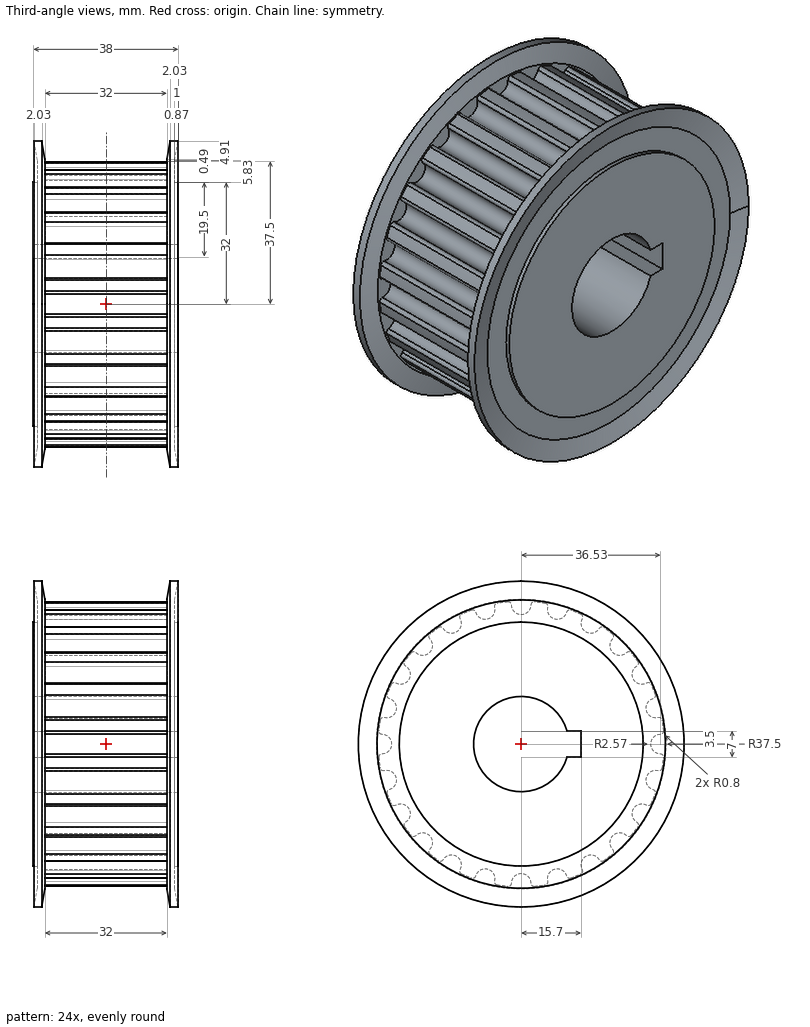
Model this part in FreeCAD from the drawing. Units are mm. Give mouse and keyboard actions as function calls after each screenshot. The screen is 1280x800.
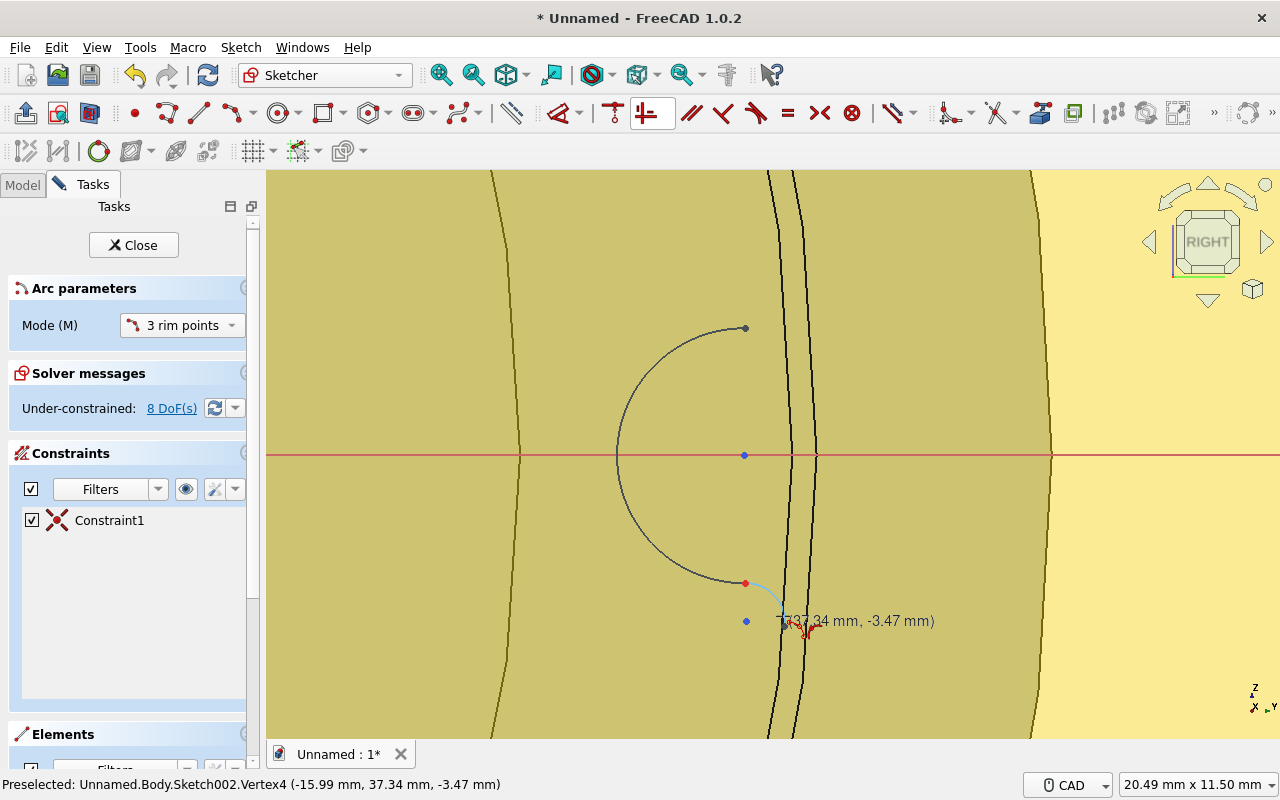
click(785, 284)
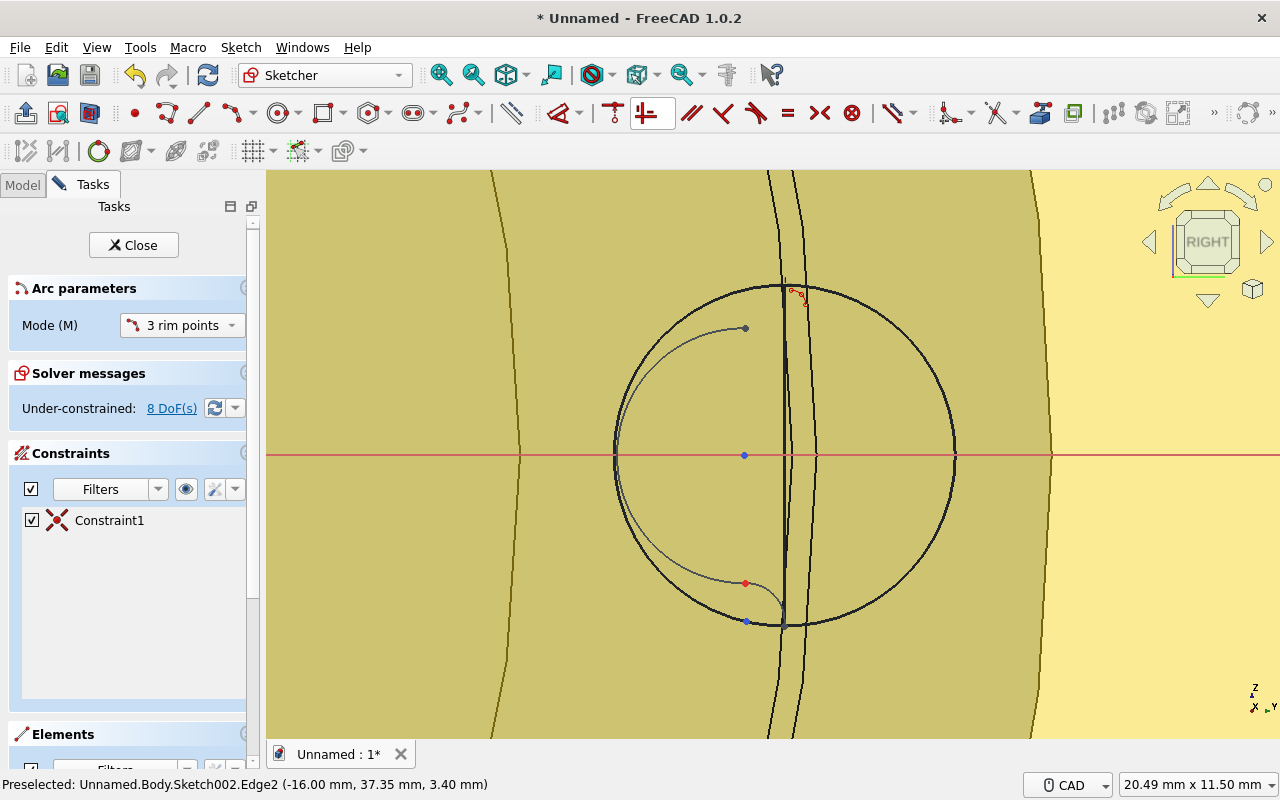
scroll(792, 489, up, 4)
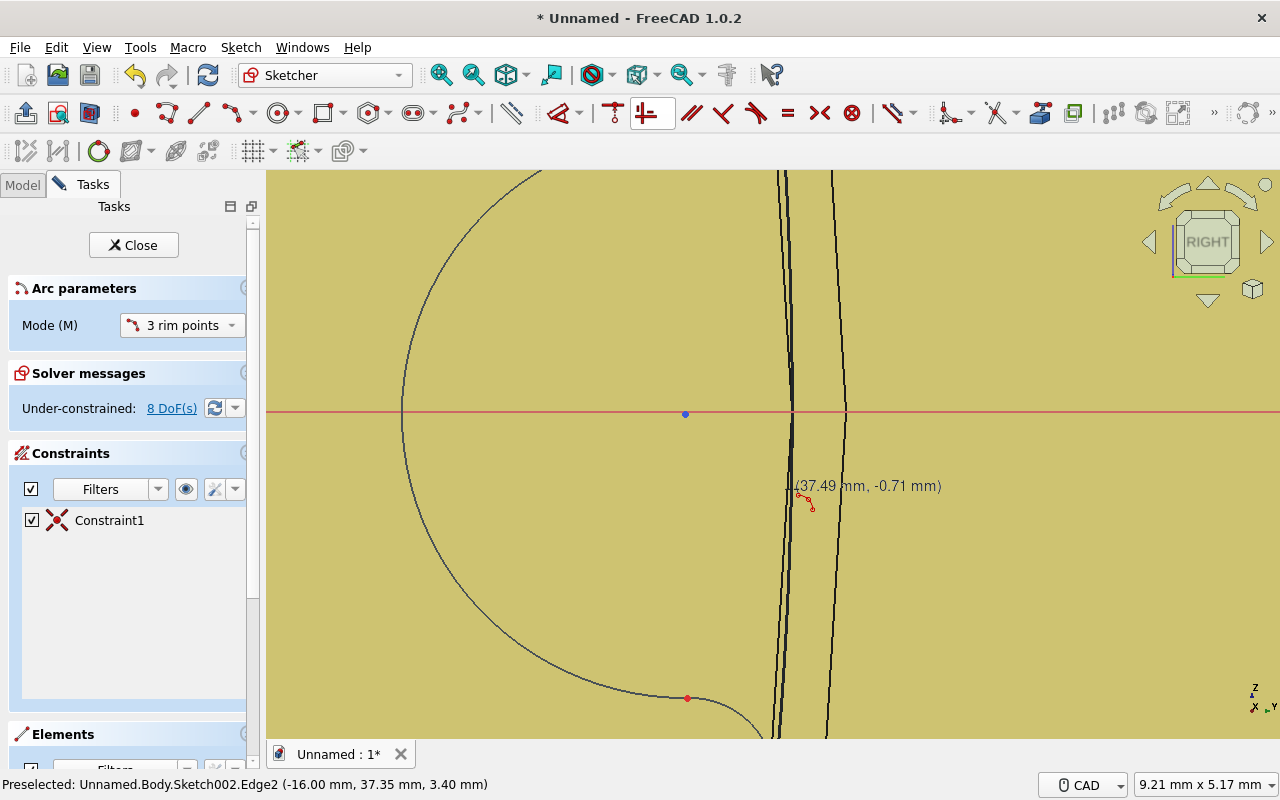
click(791, 488)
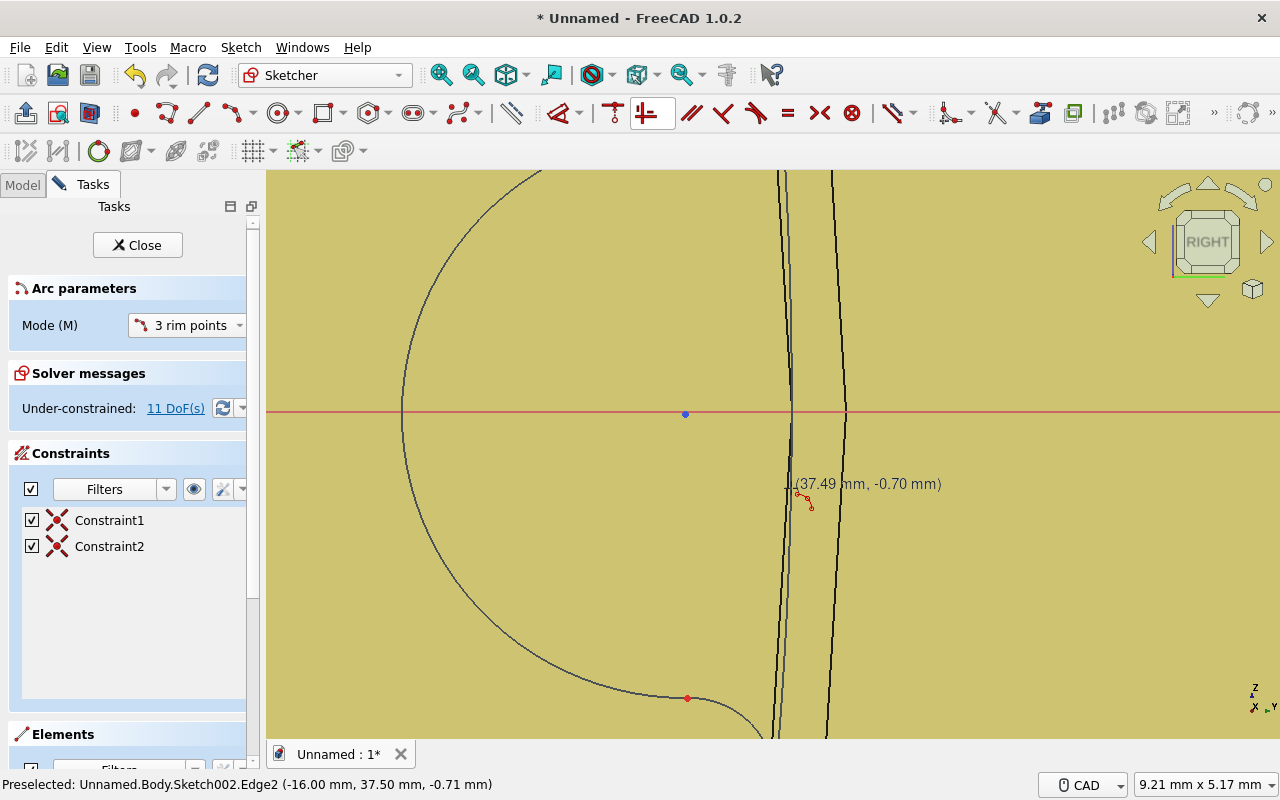
scroll(792, 489, down, 4)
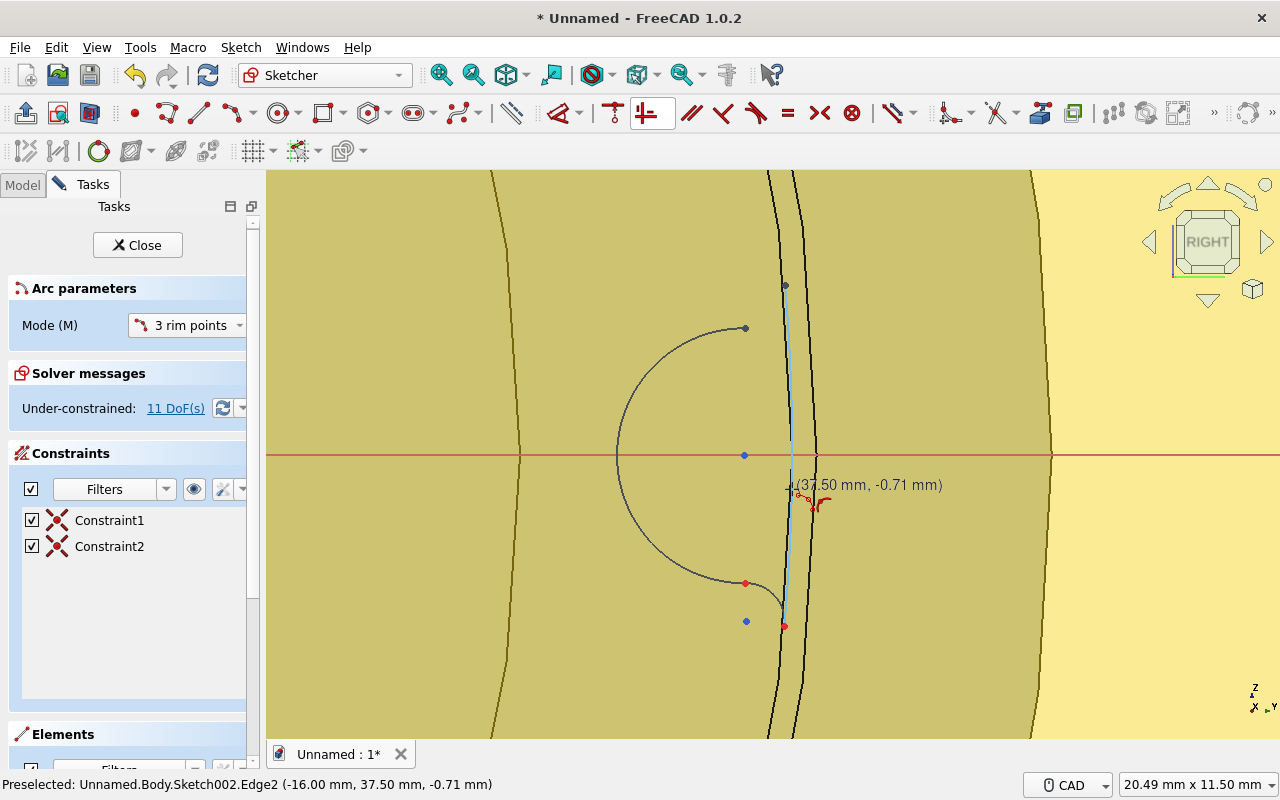
click(785, 285)
click(745, 328)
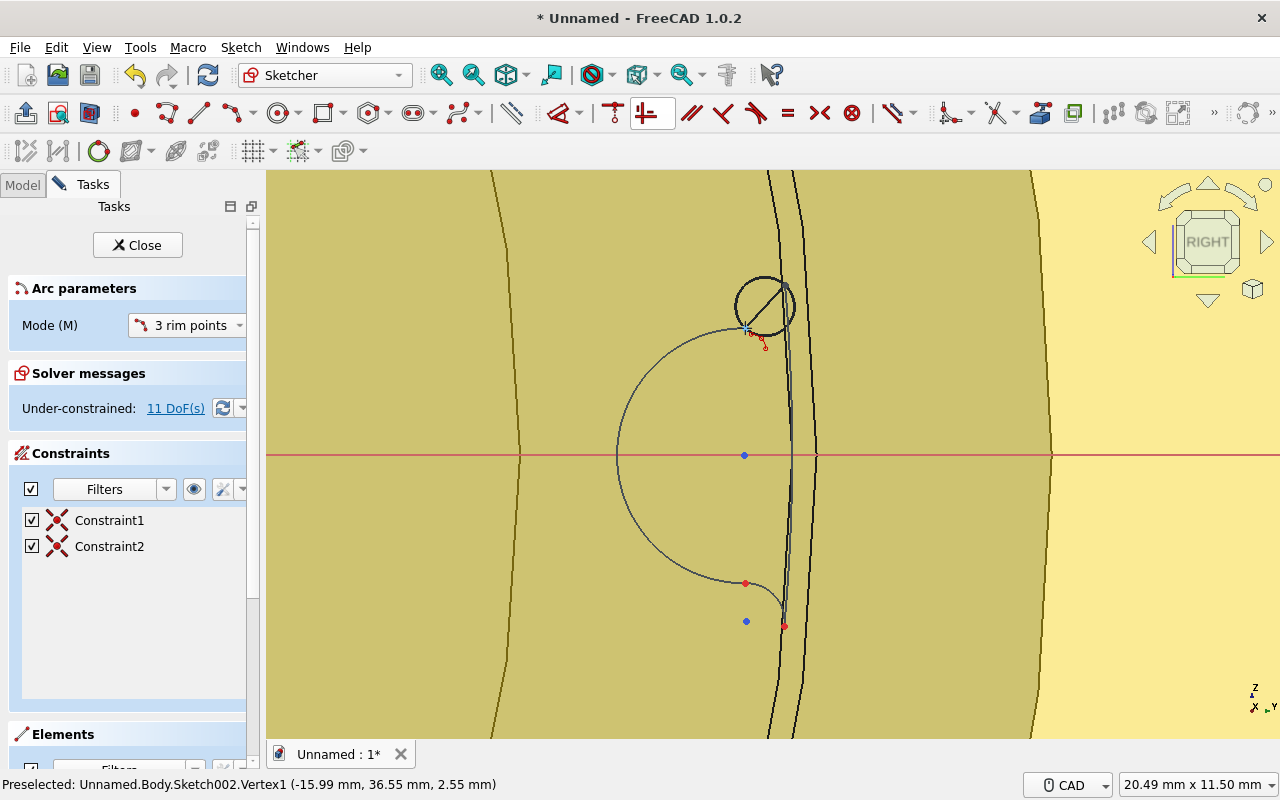
scroll(774, 315, up, 2)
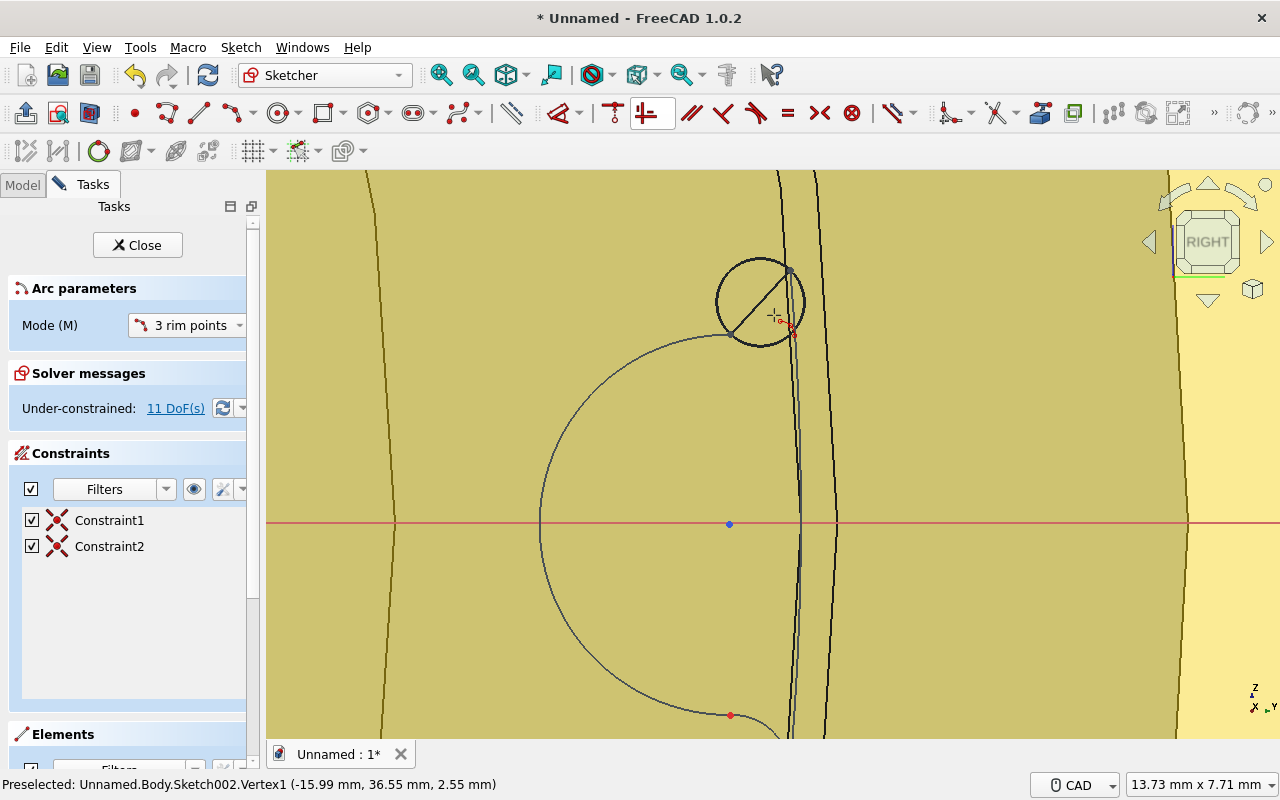
click(774, 314)
key(Escape)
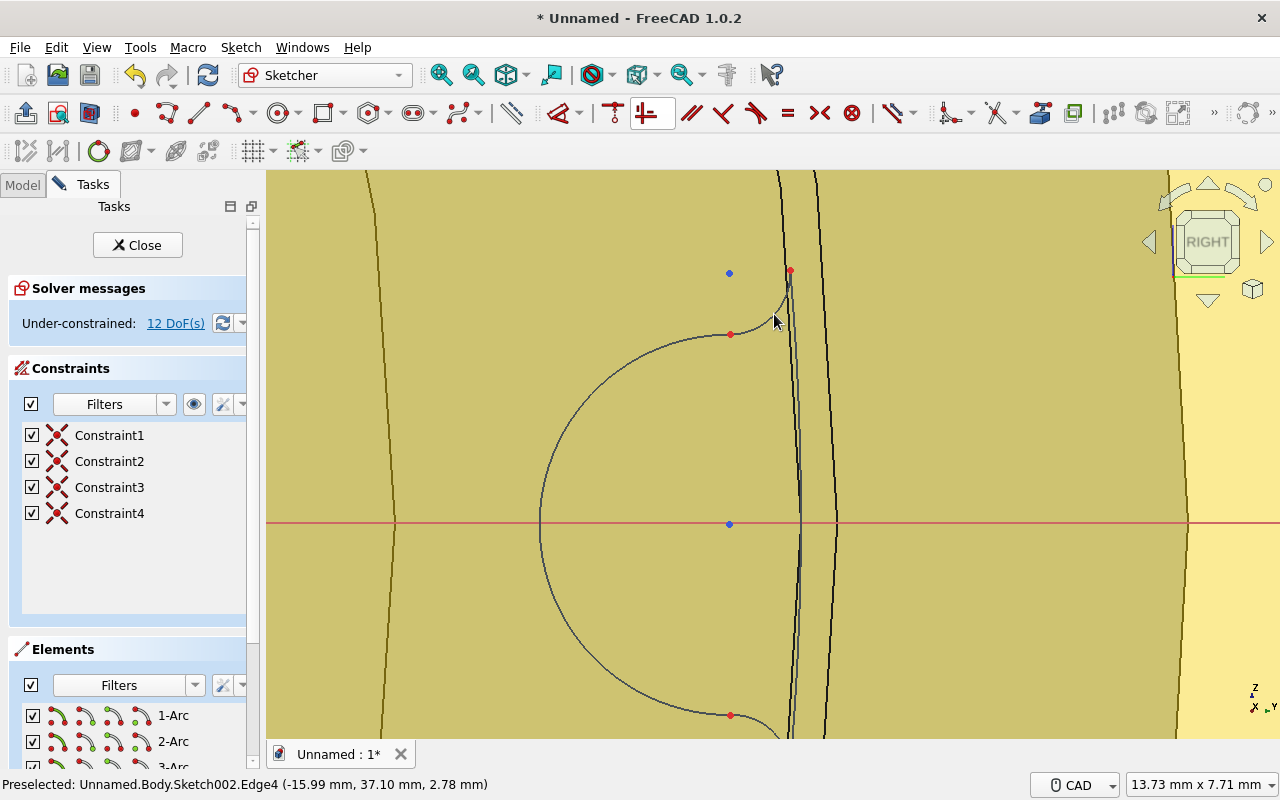
click(576, 413)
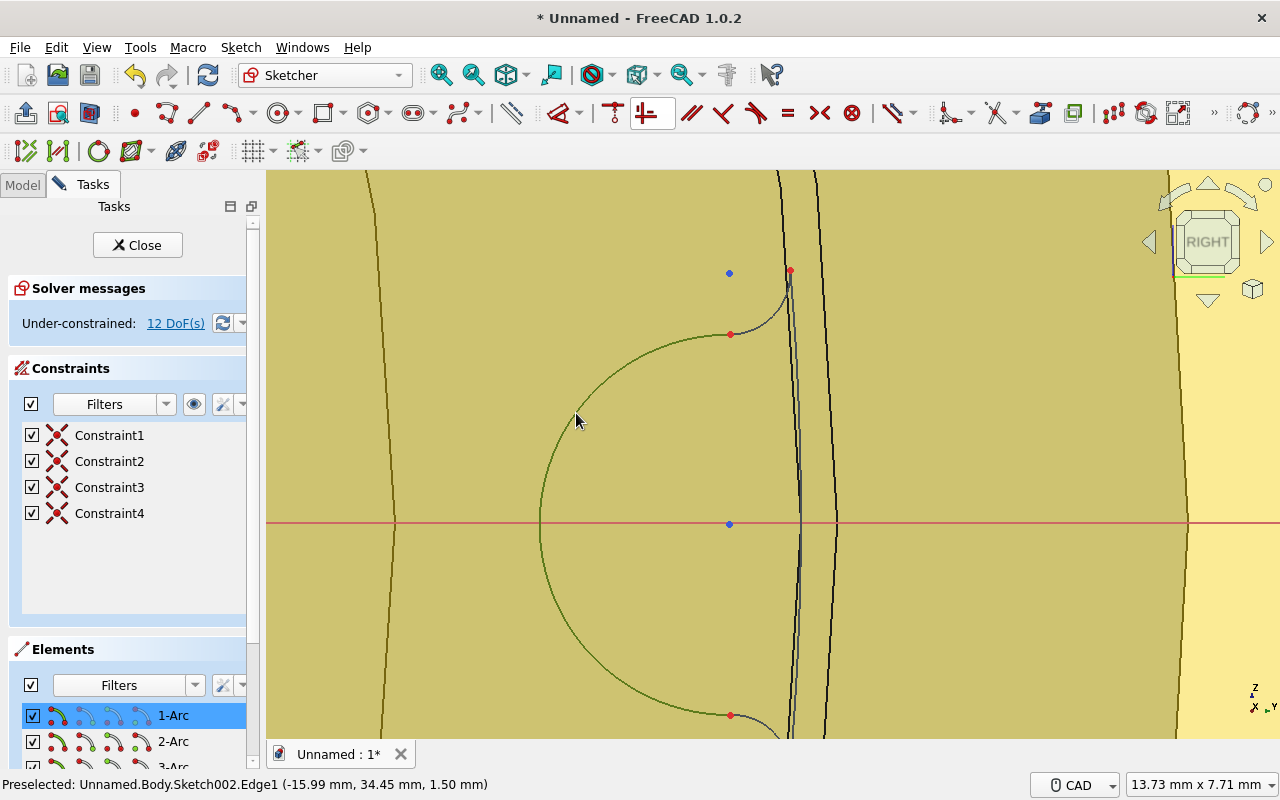
scroll(774, 315, down, 2)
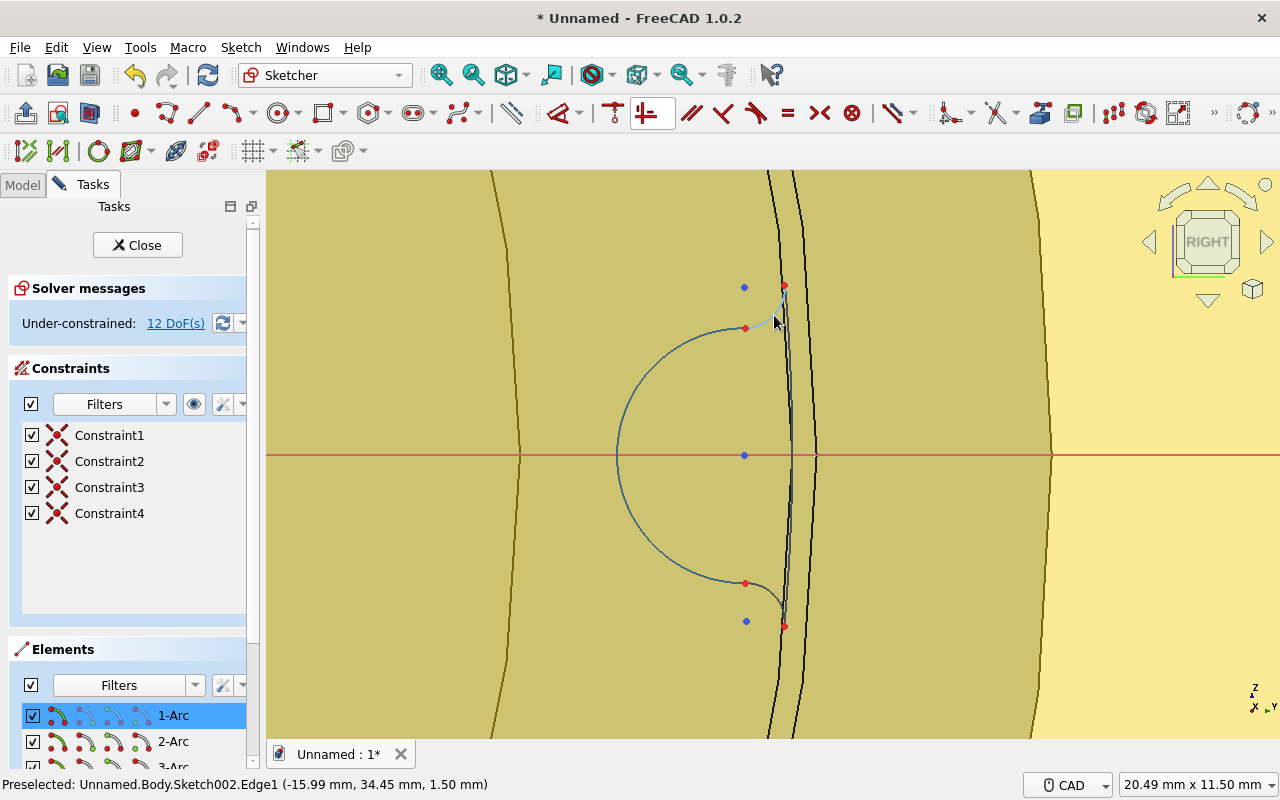
click(764, 588)